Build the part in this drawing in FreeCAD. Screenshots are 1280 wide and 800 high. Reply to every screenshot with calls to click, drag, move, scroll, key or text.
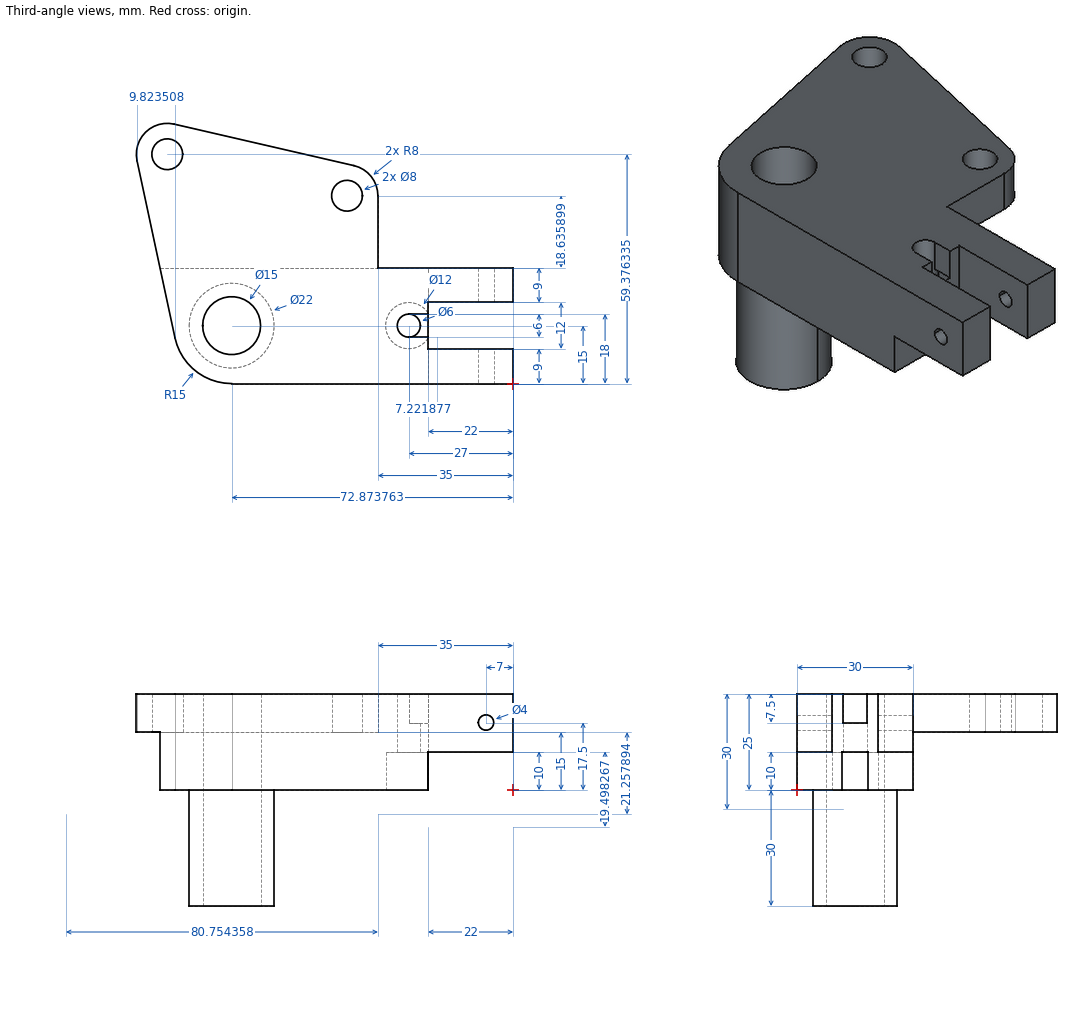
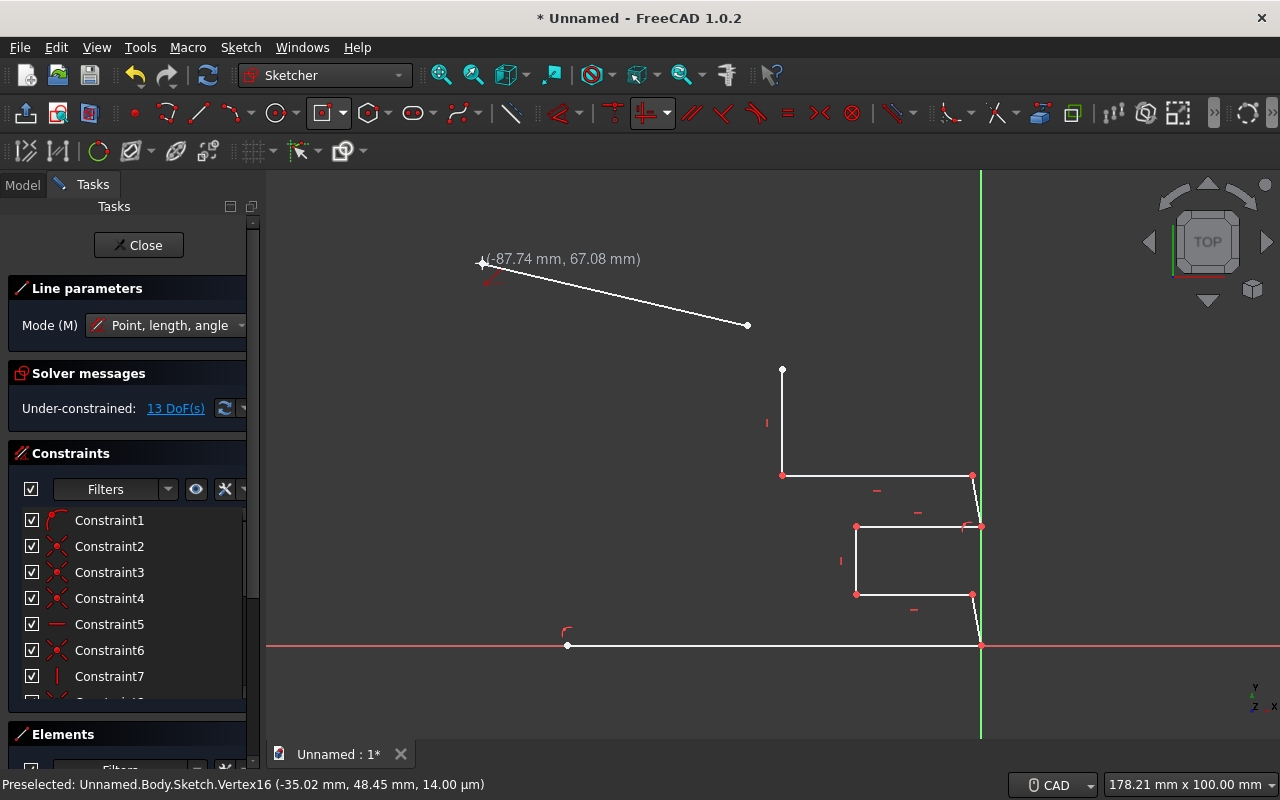
click(427, 317)
click(483, 578)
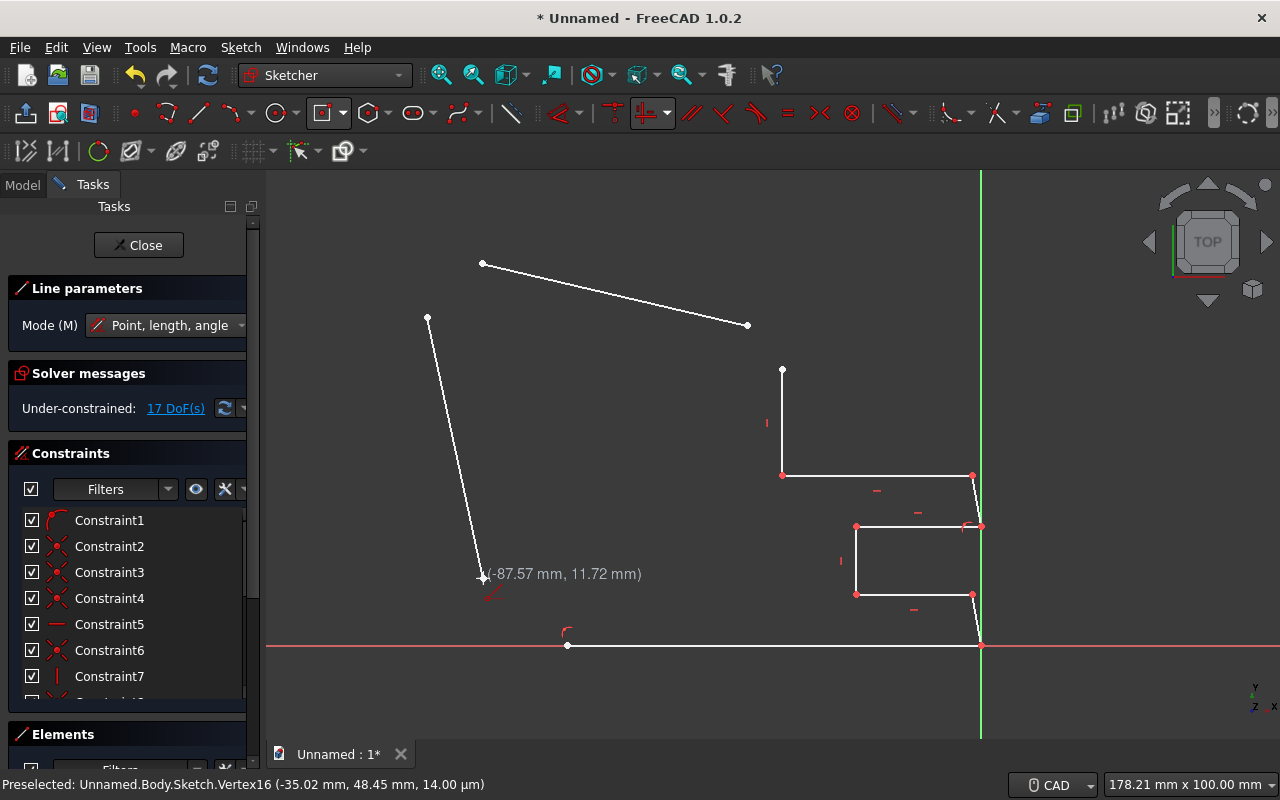
click(232, 114)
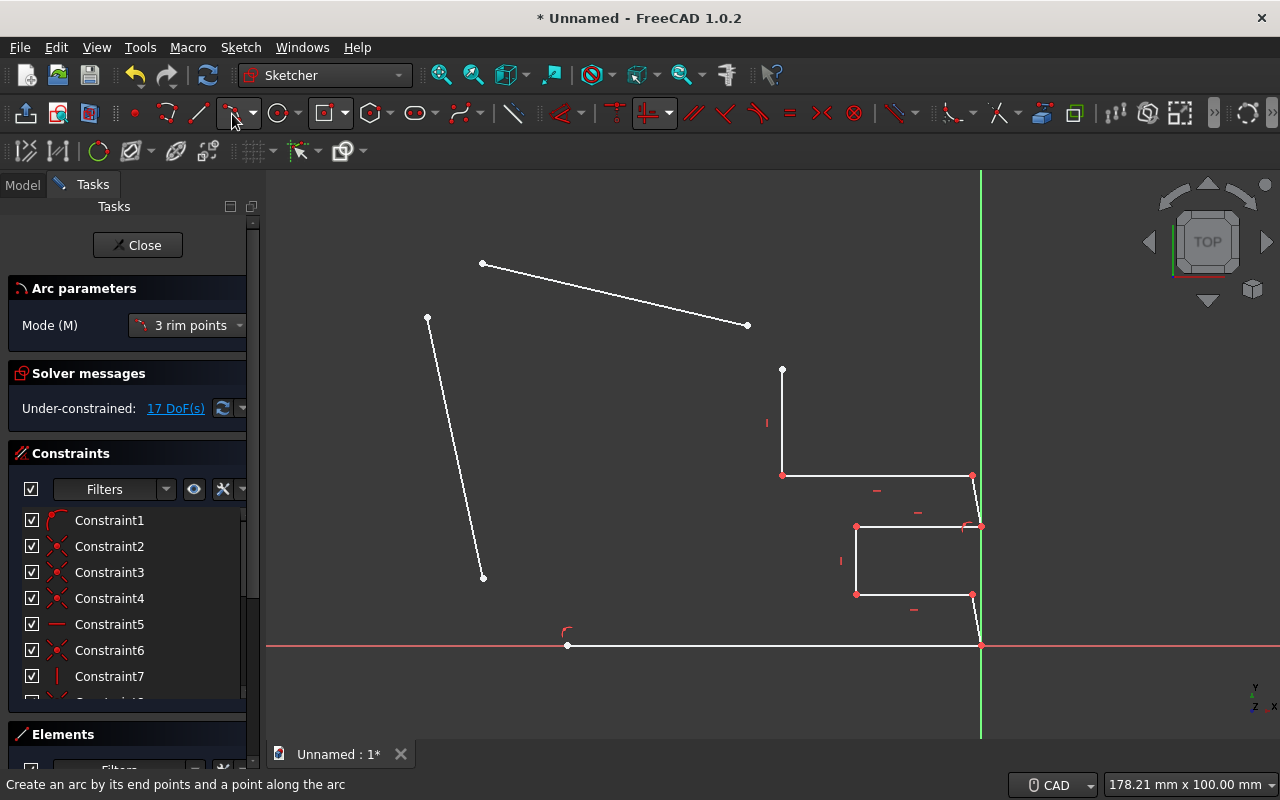
click(782, 370)
click(747, 326)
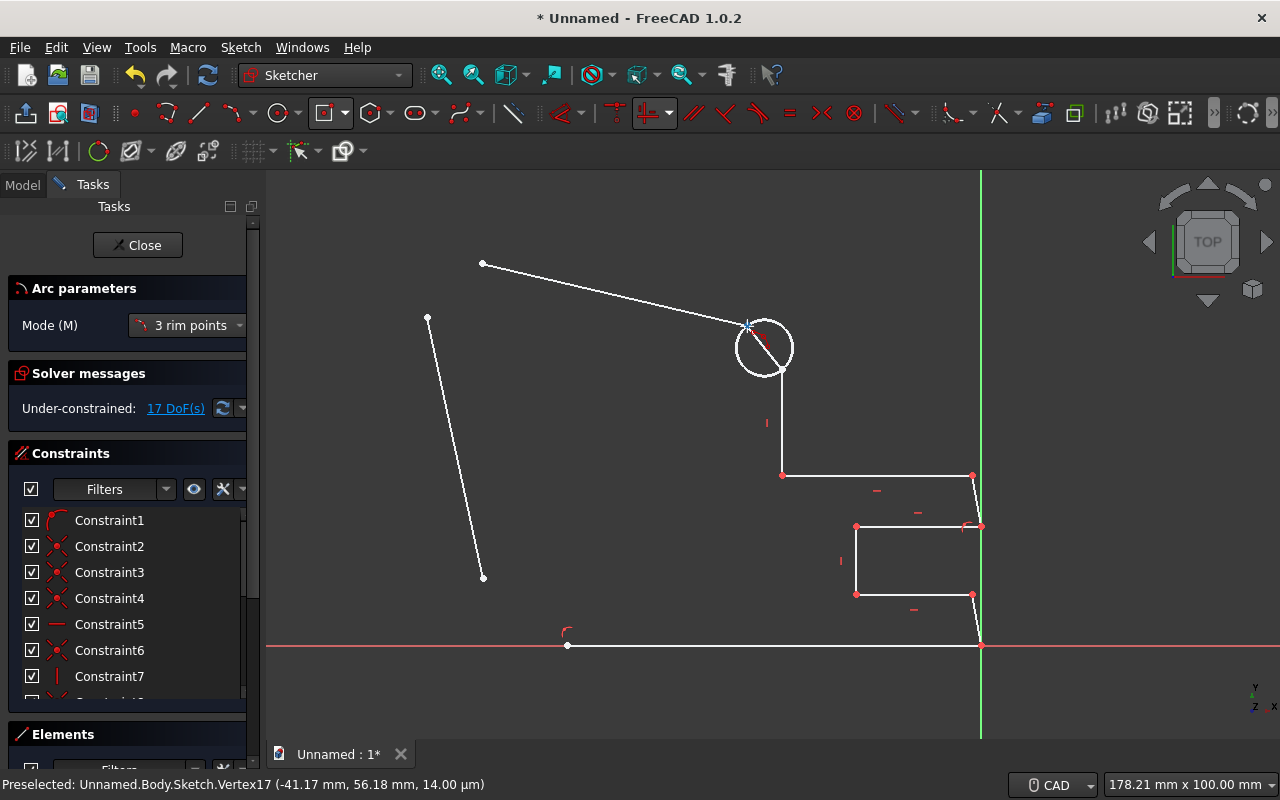
scroll(772, 341, up, 3)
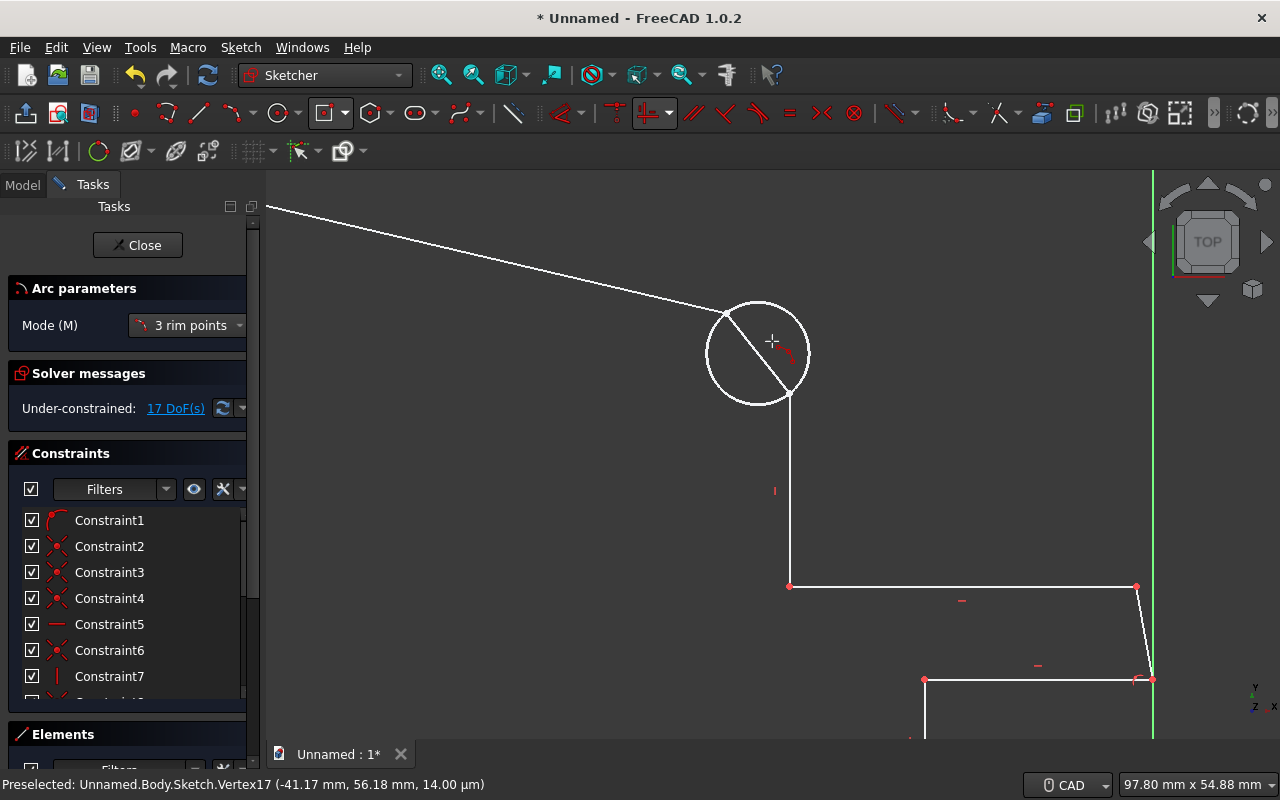
click(772, 340)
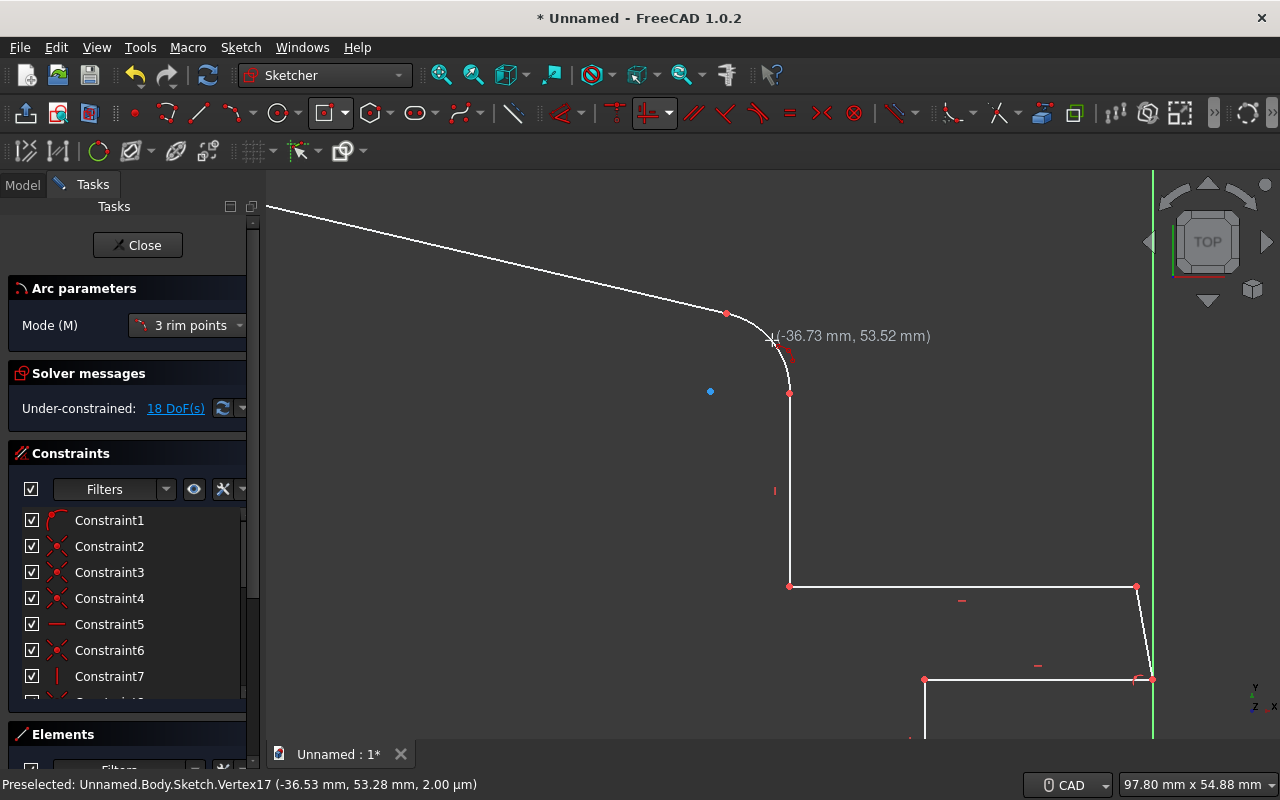
scroll(773, 341, down, 3)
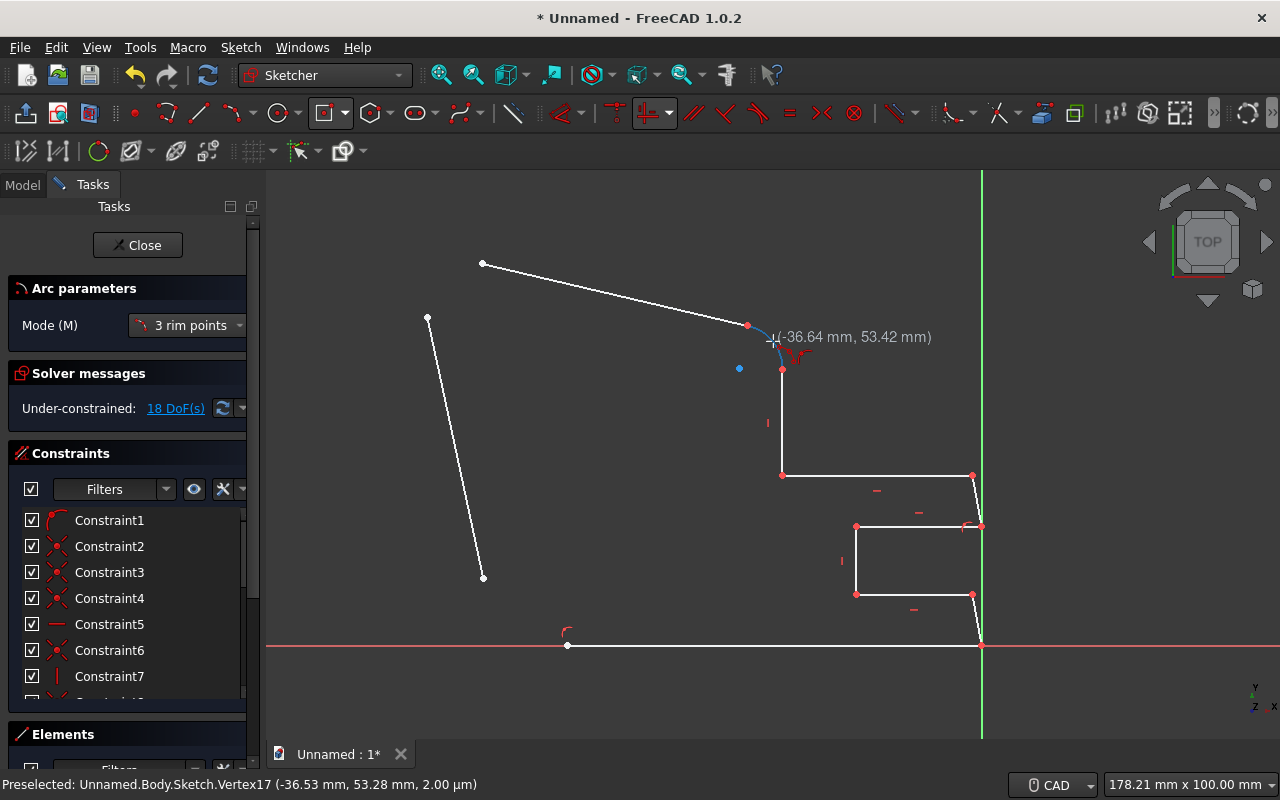
click(482, 264)
click(427, 318)
click(440, 275)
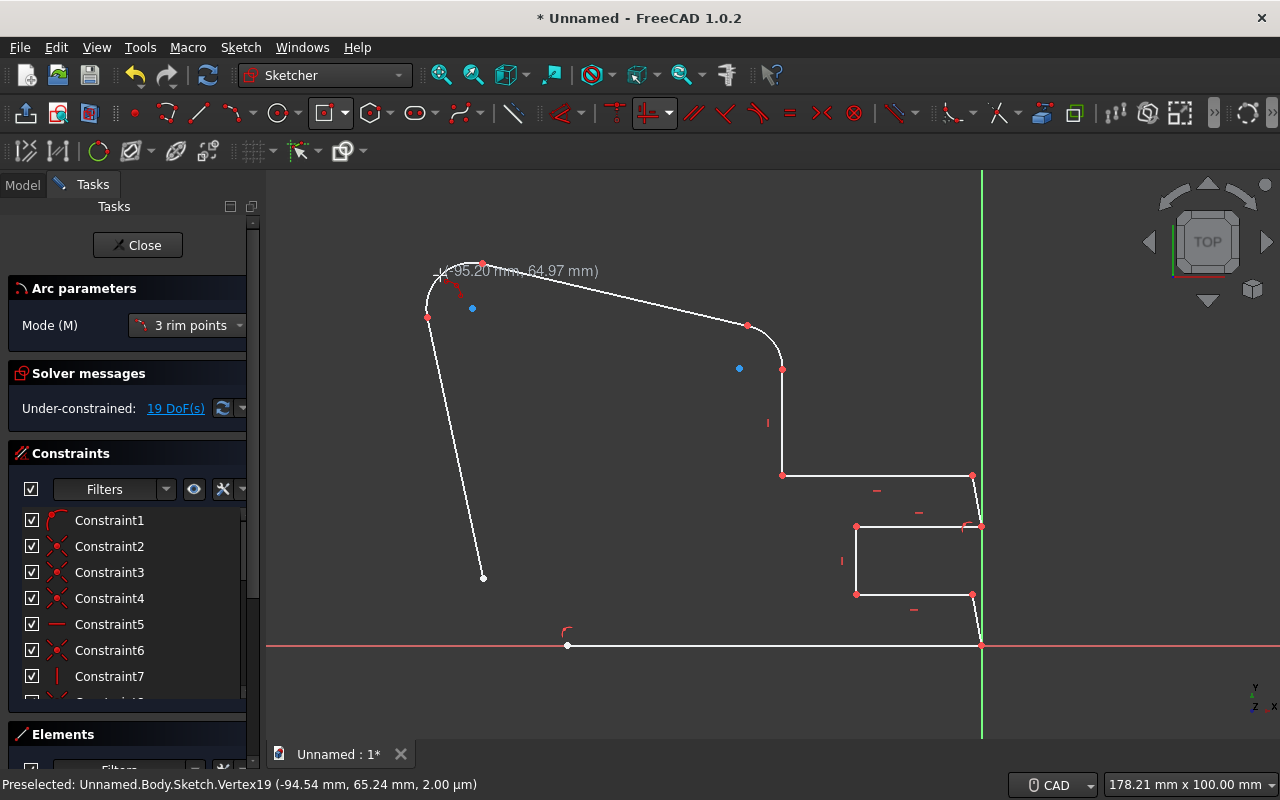
click(483, 579)
click(567, 646)
click(513, 627)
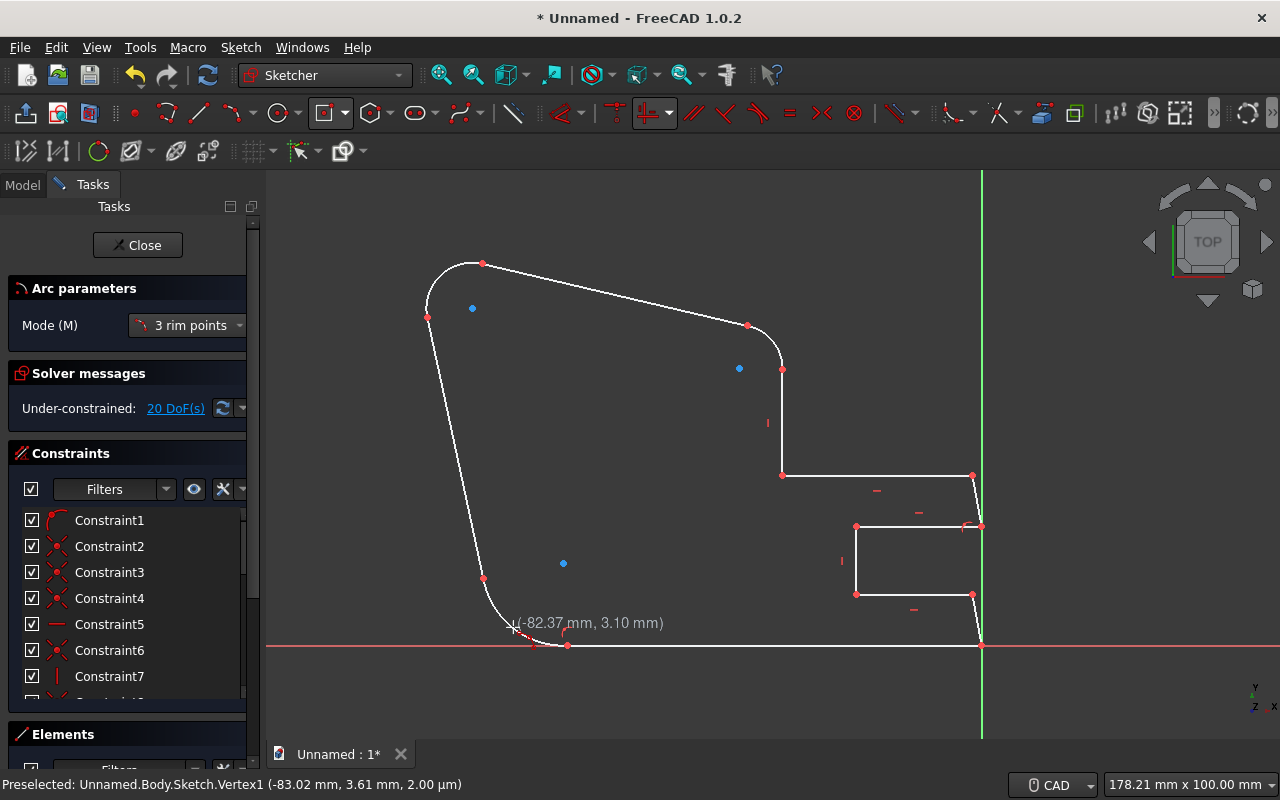
click(278, 114)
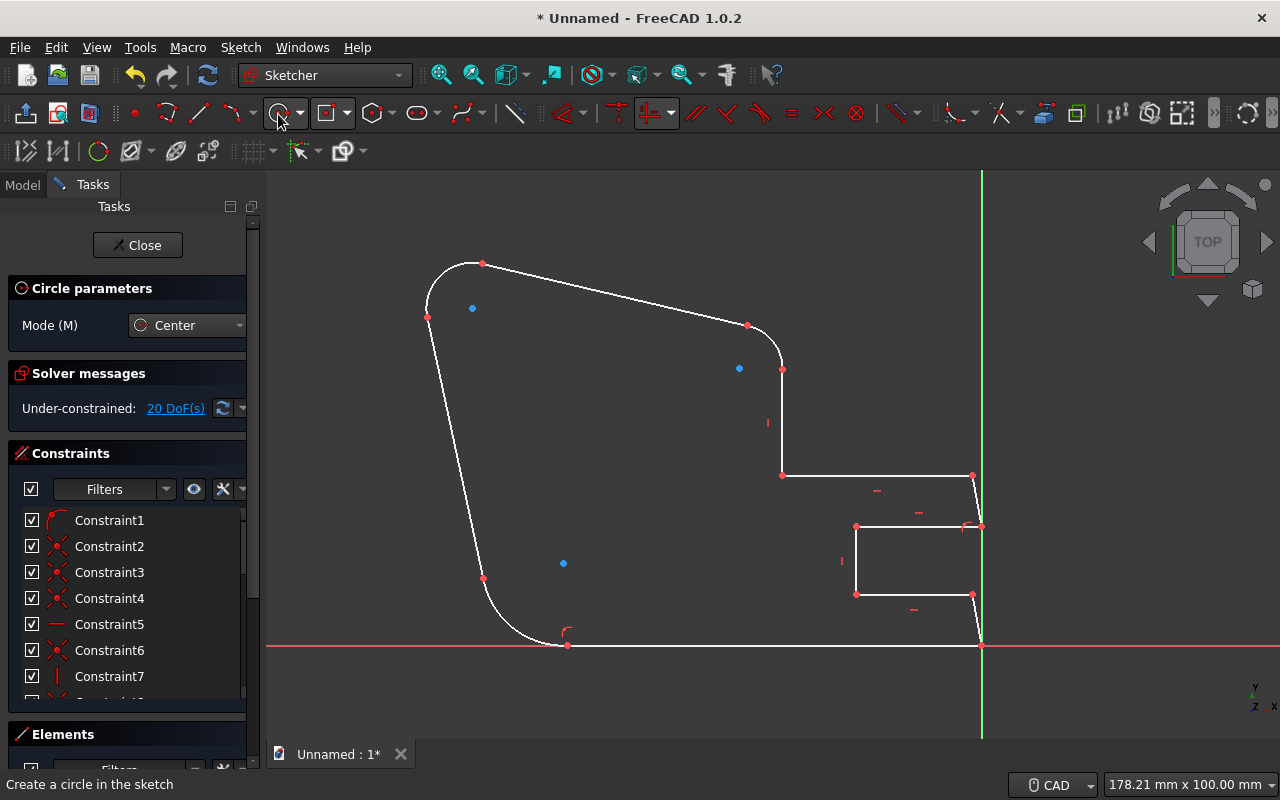
click(737, 369)
click(753, 353)